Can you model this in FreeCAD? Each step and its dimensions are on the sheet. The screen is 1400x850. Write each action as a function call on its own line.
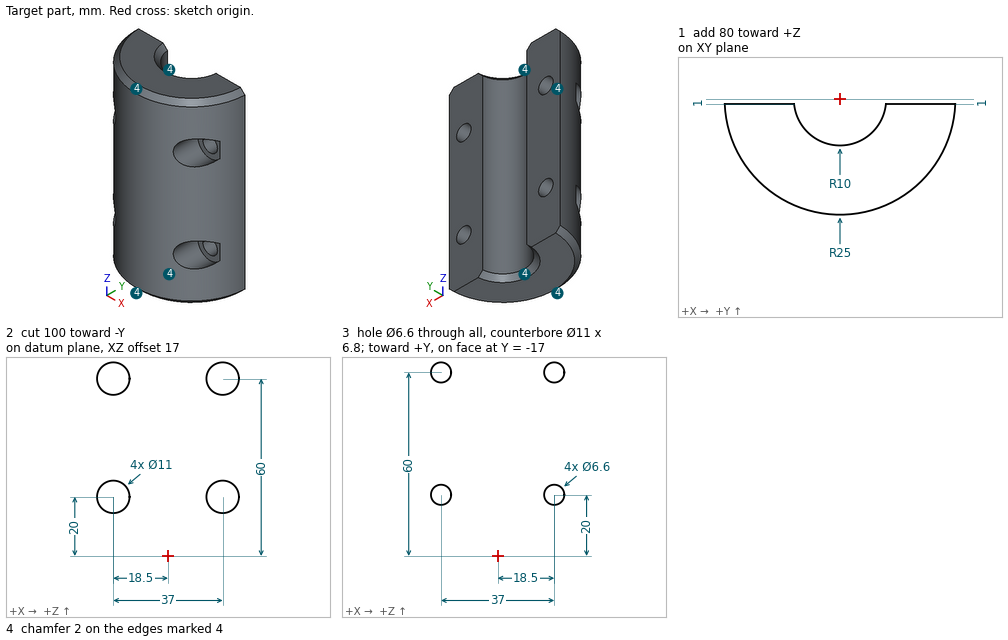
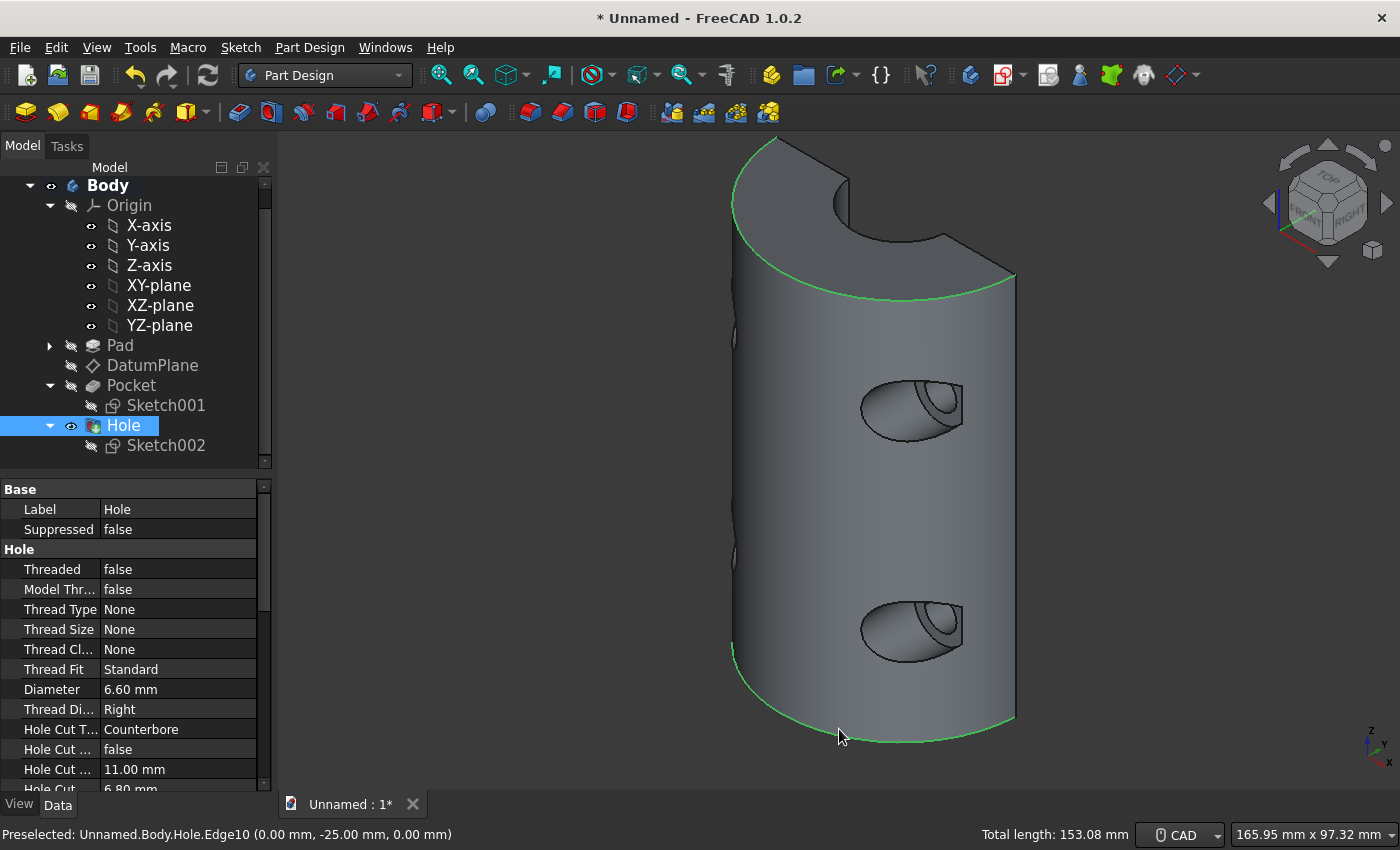
click(837, 190, ctrl)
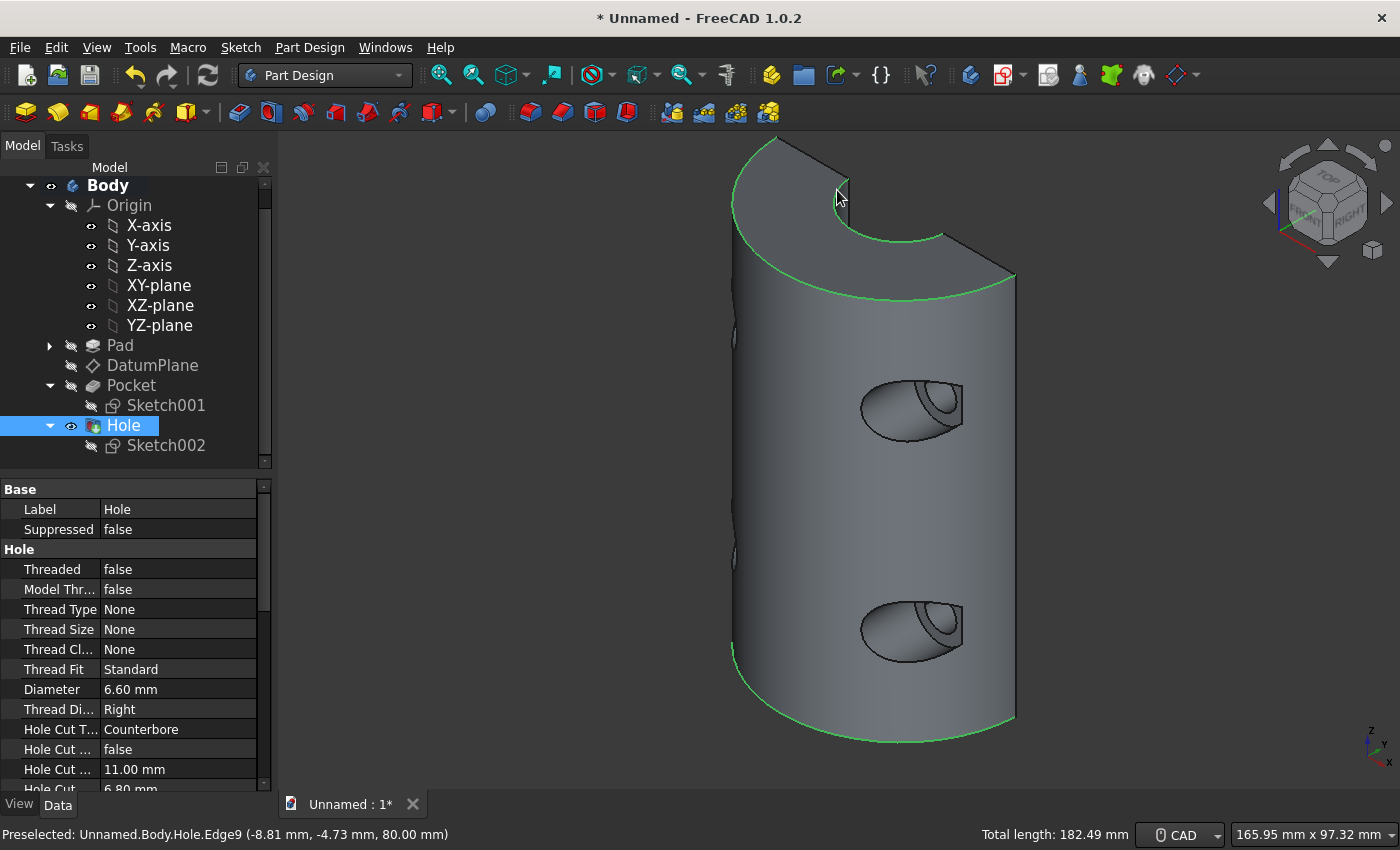
key(2)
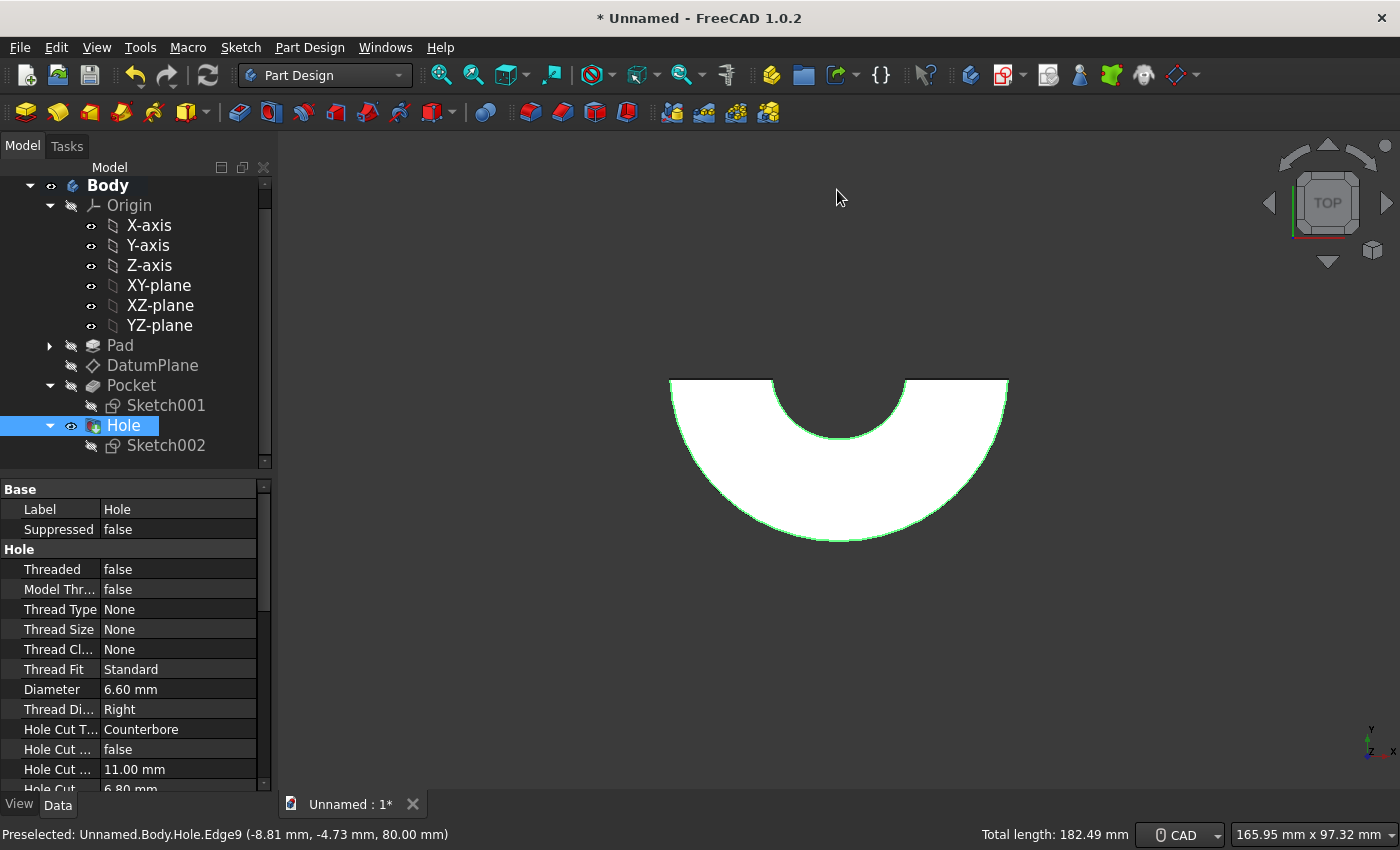
click(442, 76)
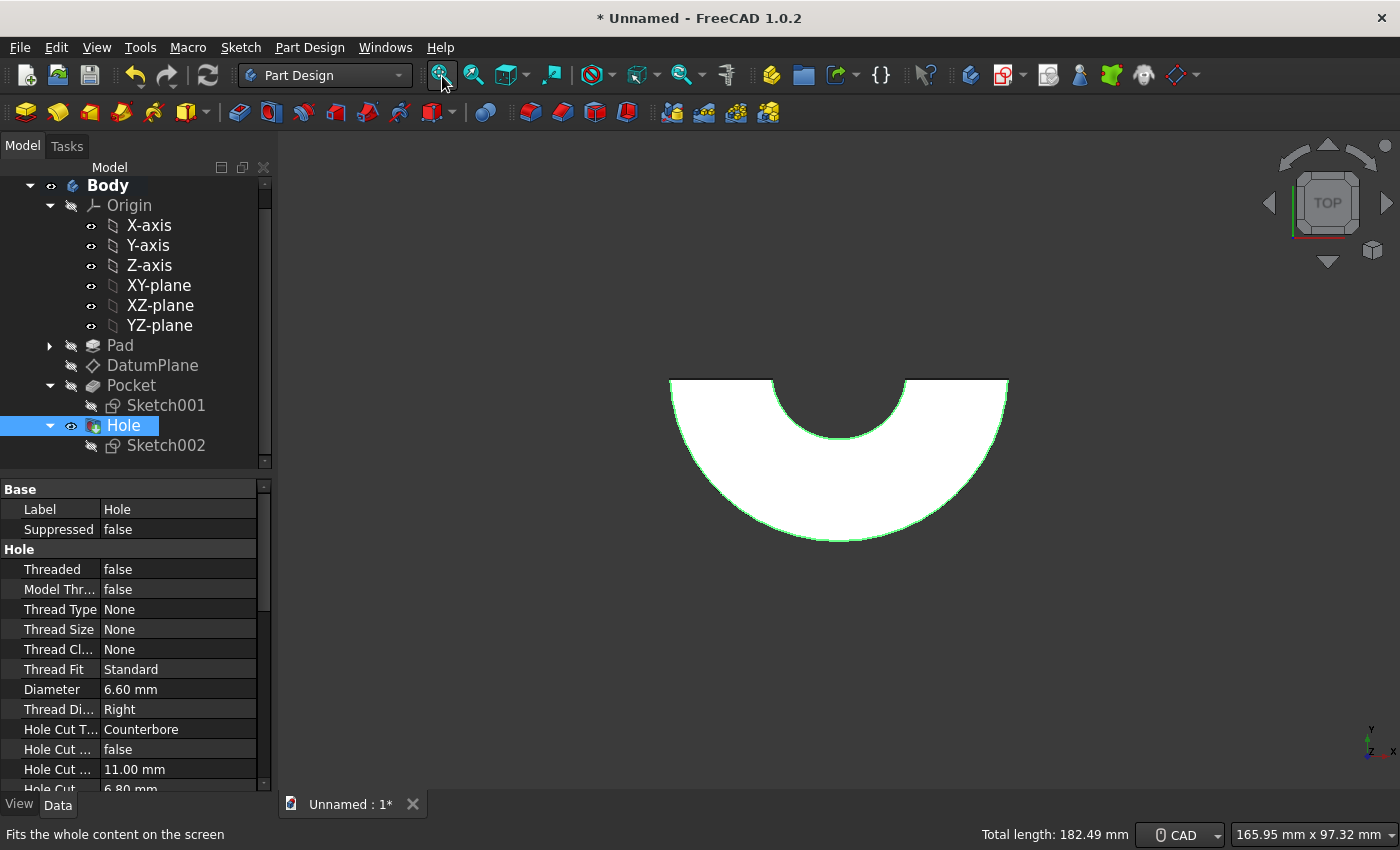
key(1)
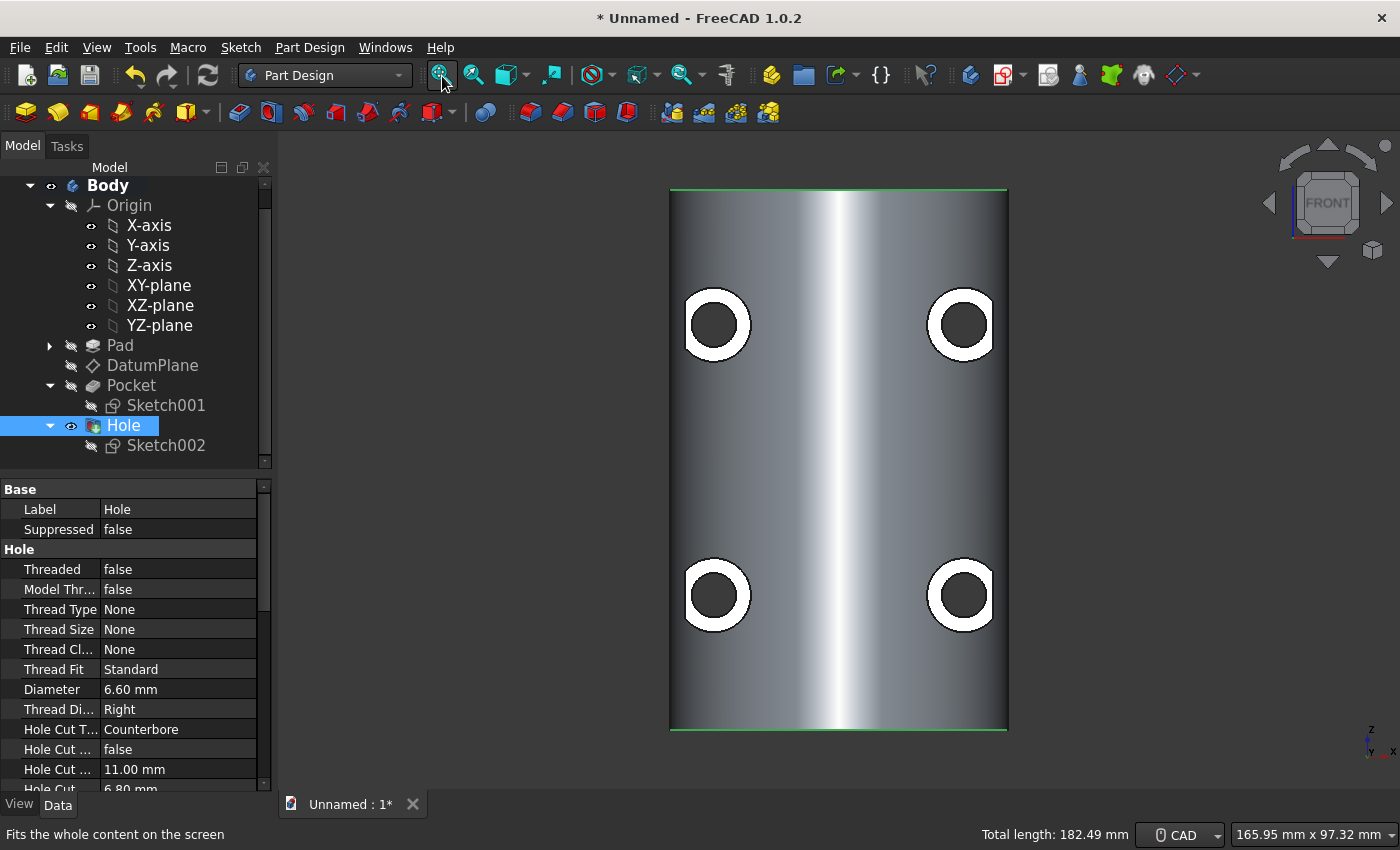
key(3)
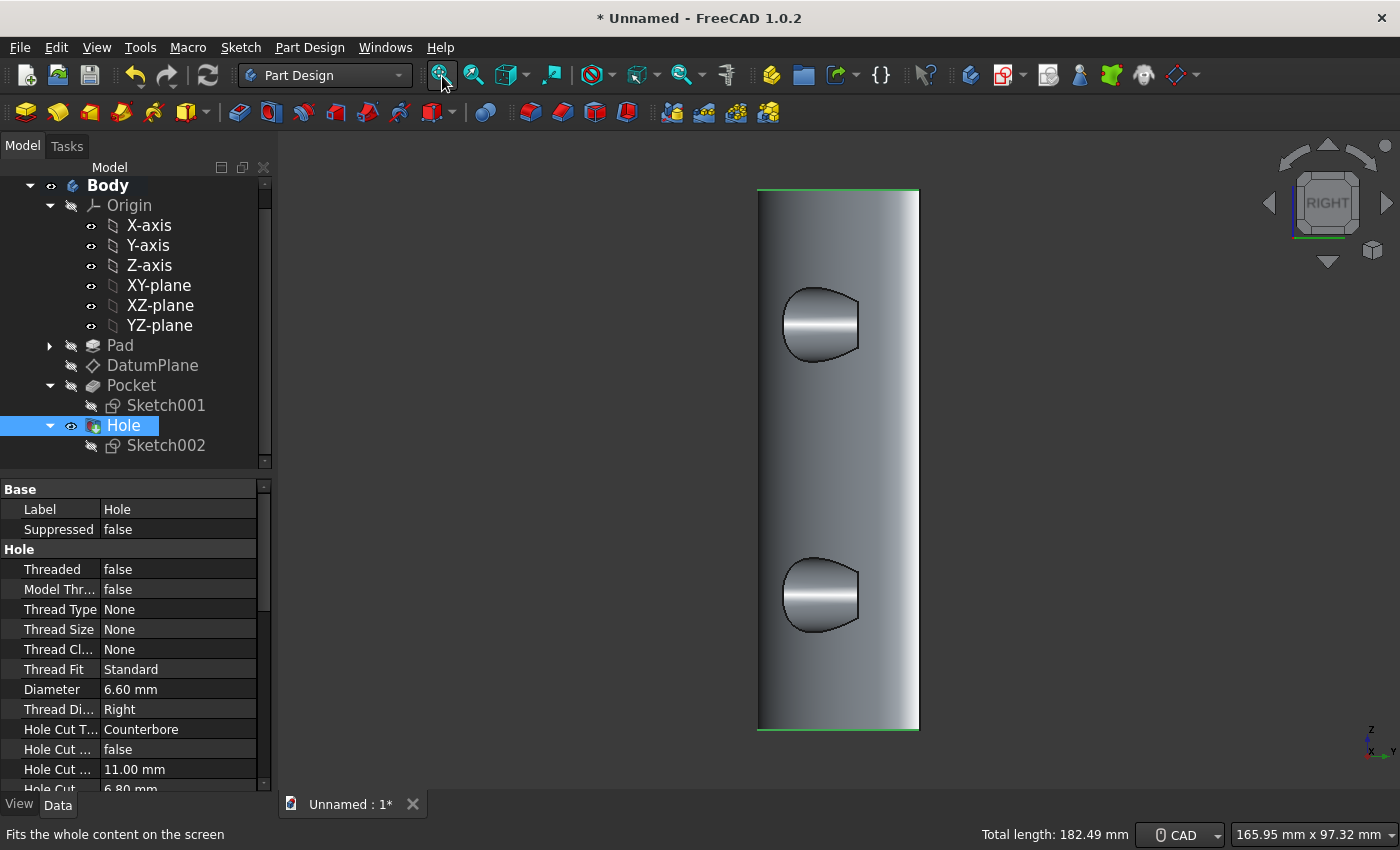
key(5)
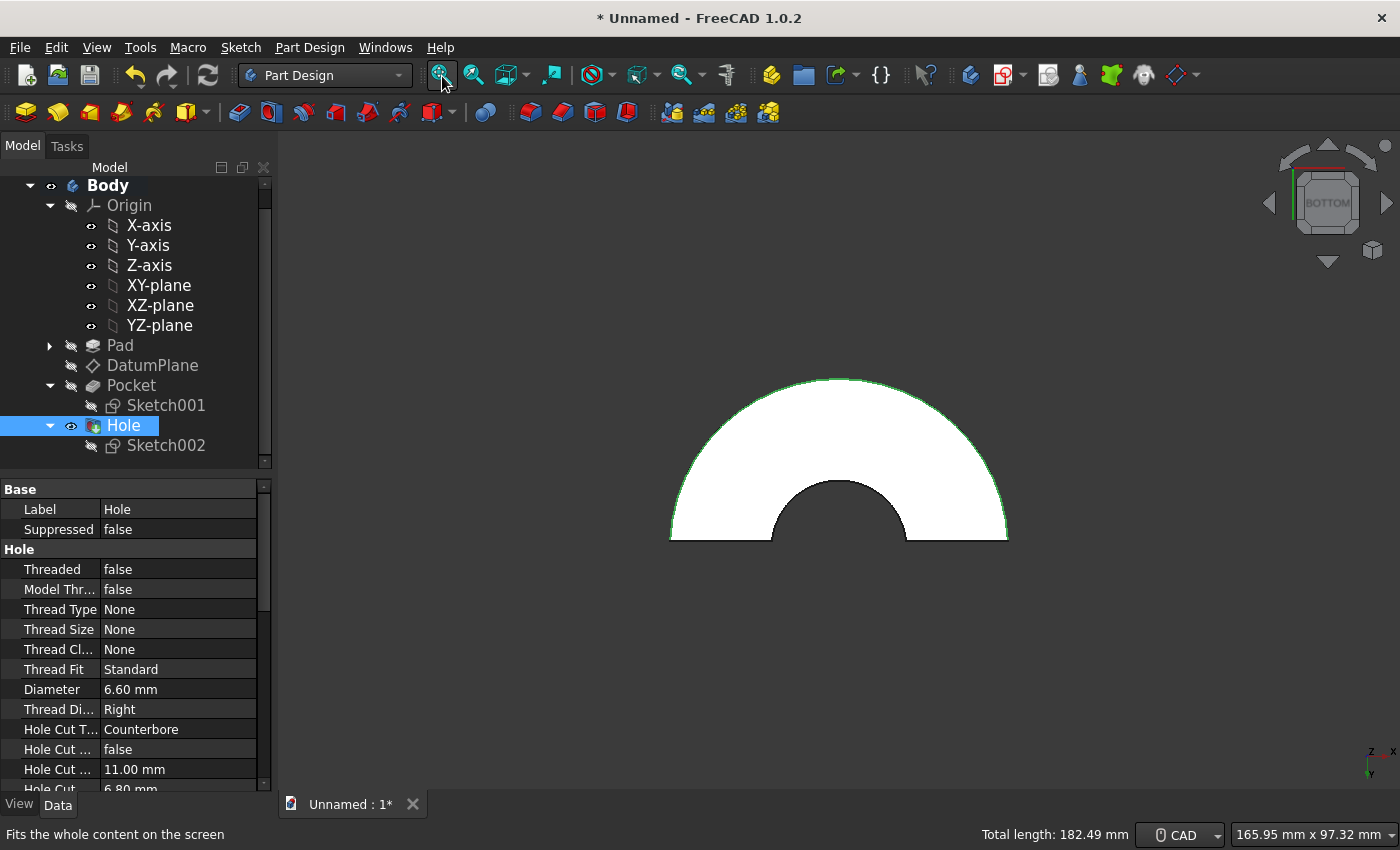
click(442, 76)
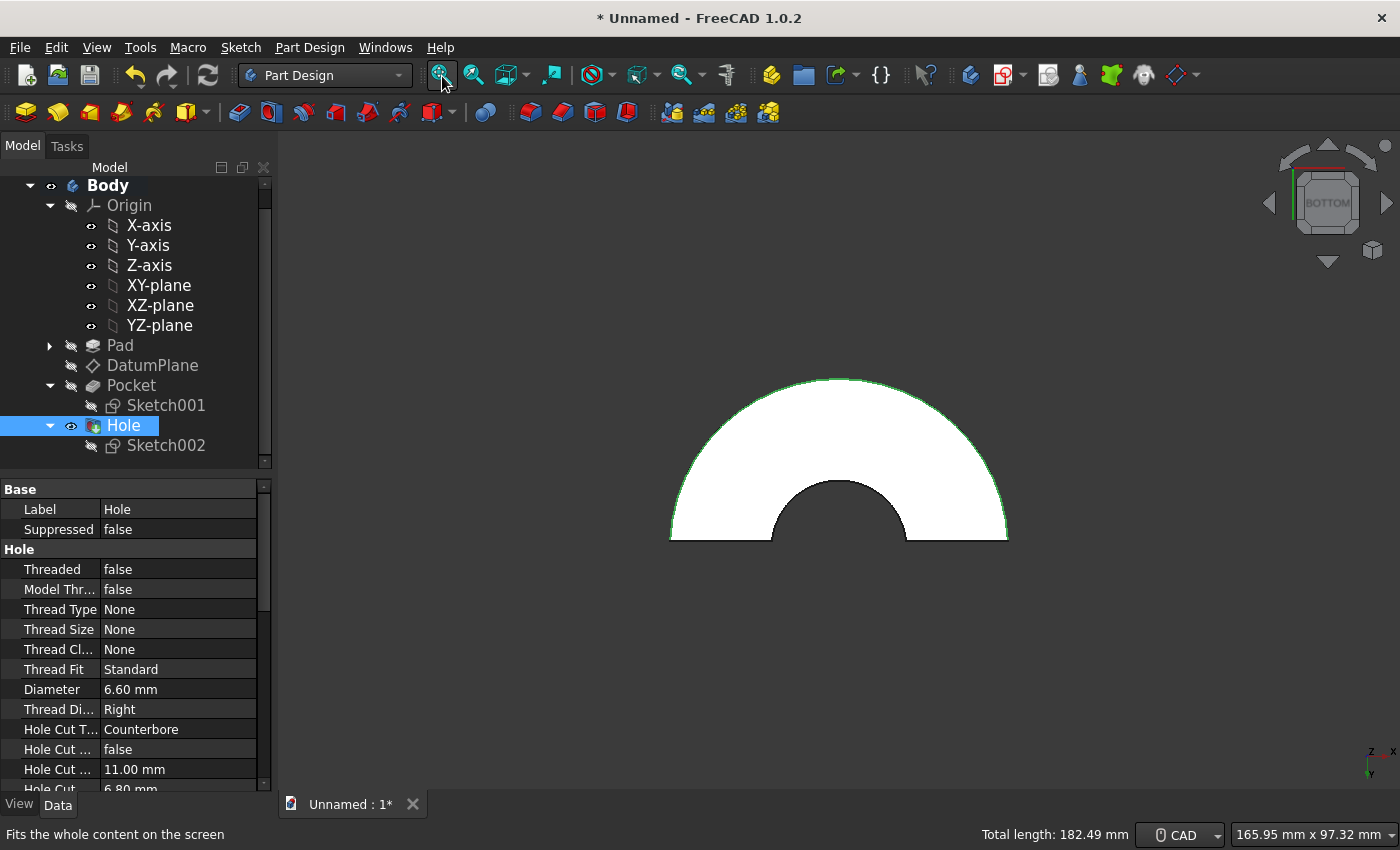
click(839, 479, ctrl)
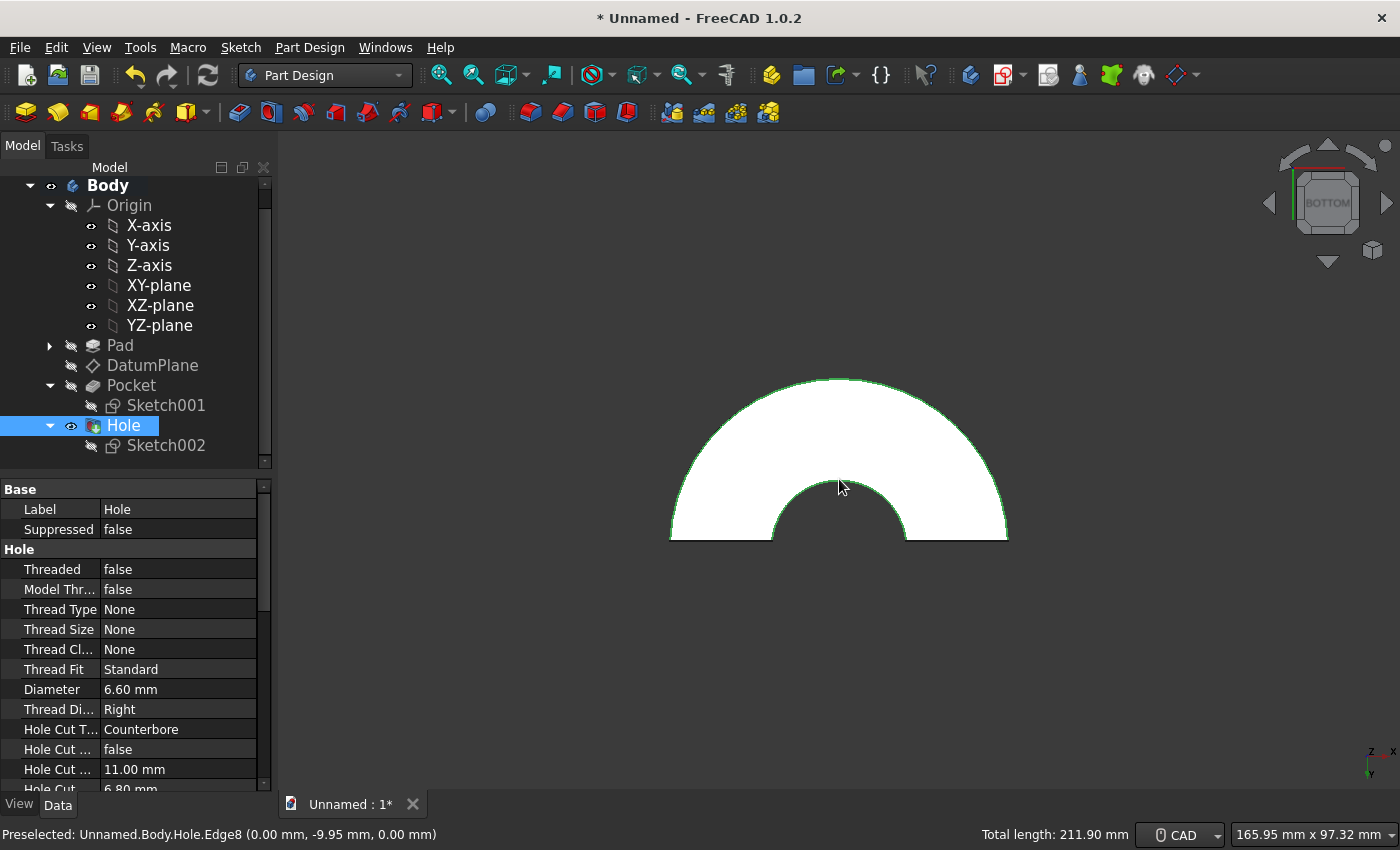
click(564, 112)